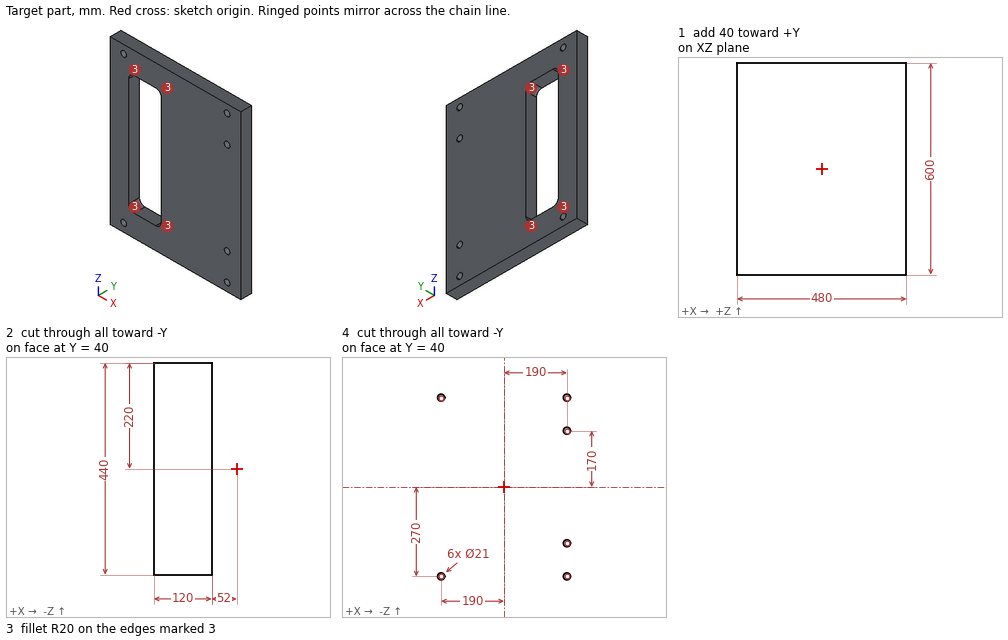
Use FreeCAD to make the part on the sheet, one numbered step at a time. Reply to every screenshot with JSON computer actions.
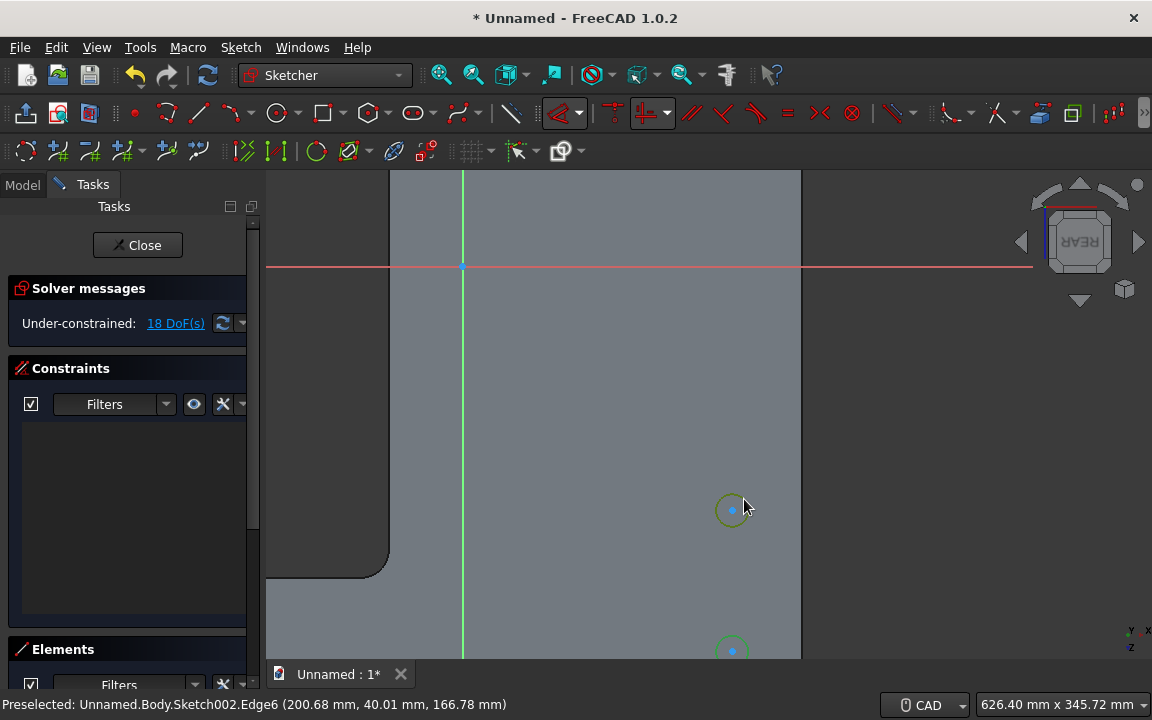
{"action": "left_click", "coordinate": [788, 114]}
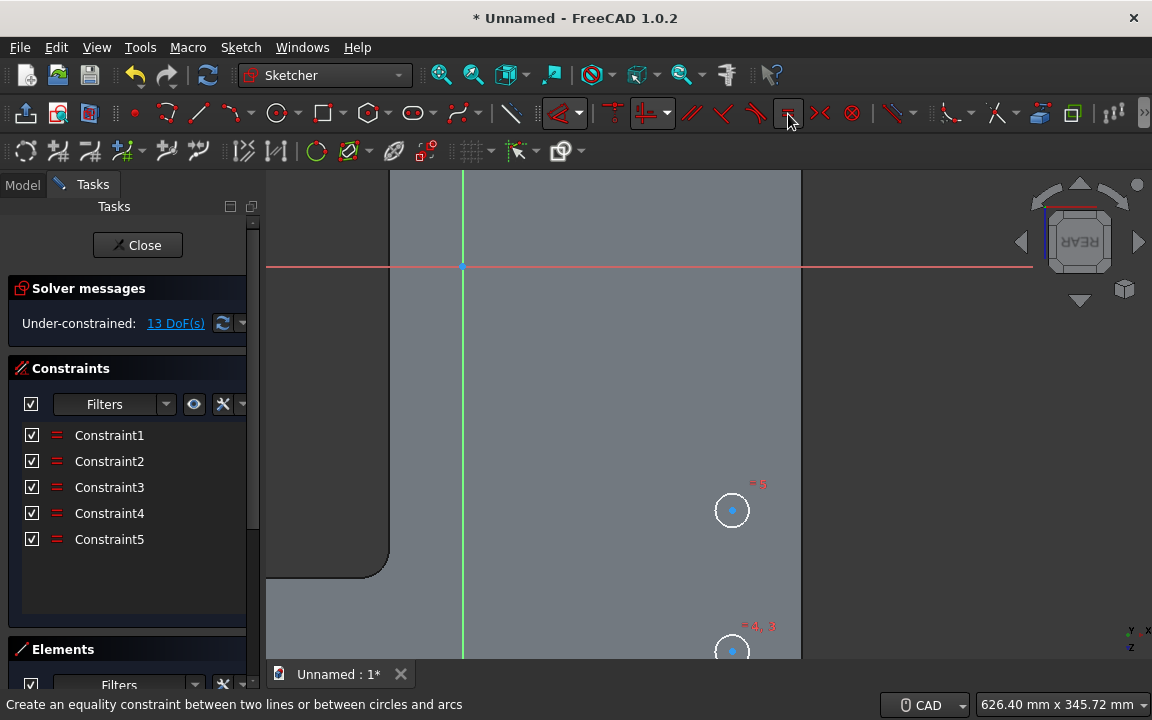
{"action": "scroll", "coordinate": [744, 500], "scroll_direction": "down", "scroll_amount": 5}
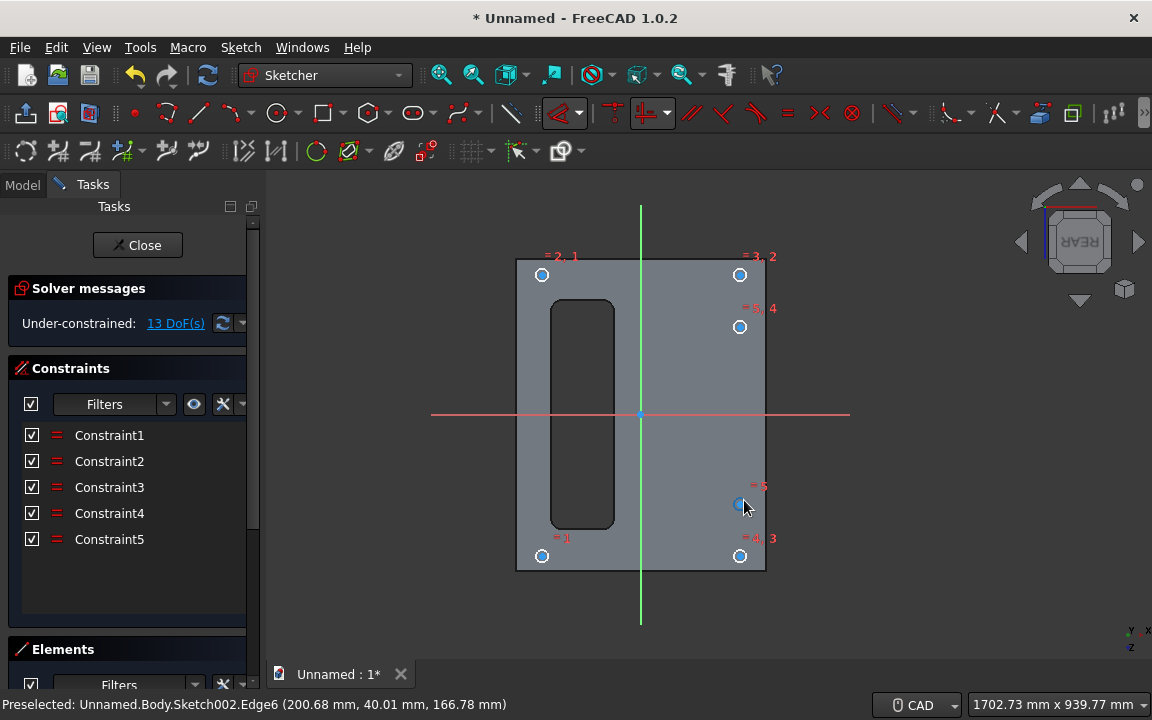
{"action": "left_click", "coordinate": [542, 556]}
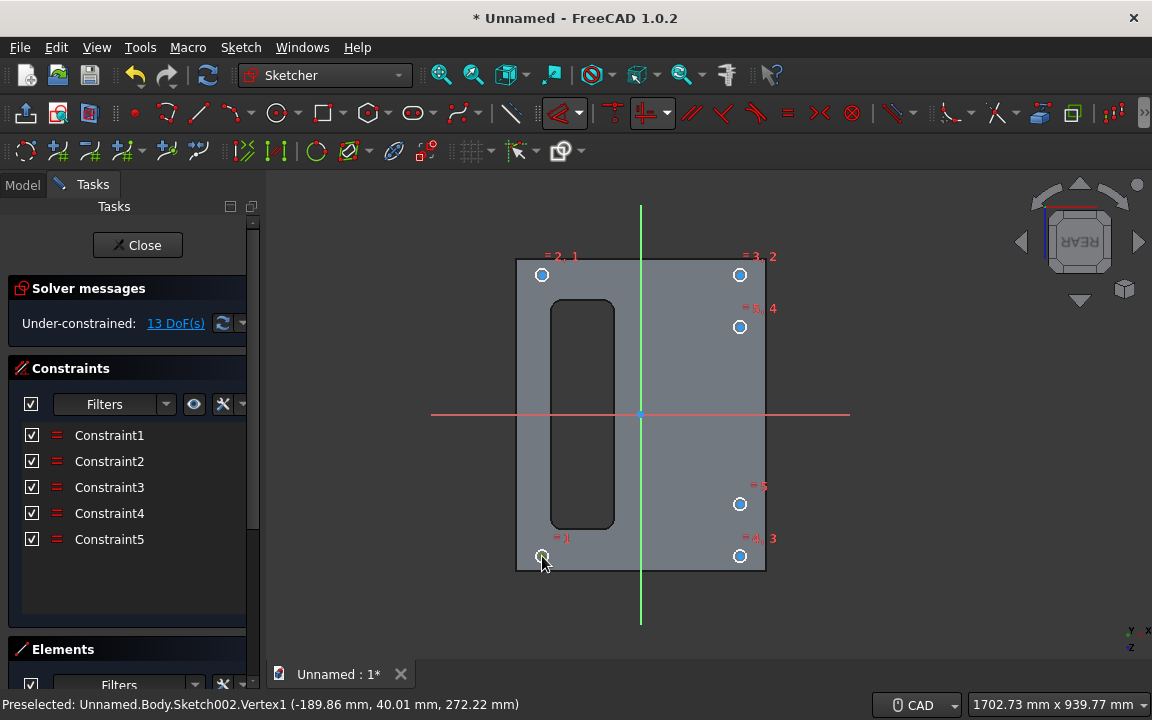
{"action": "left_click", "coordinate": [542, 275]}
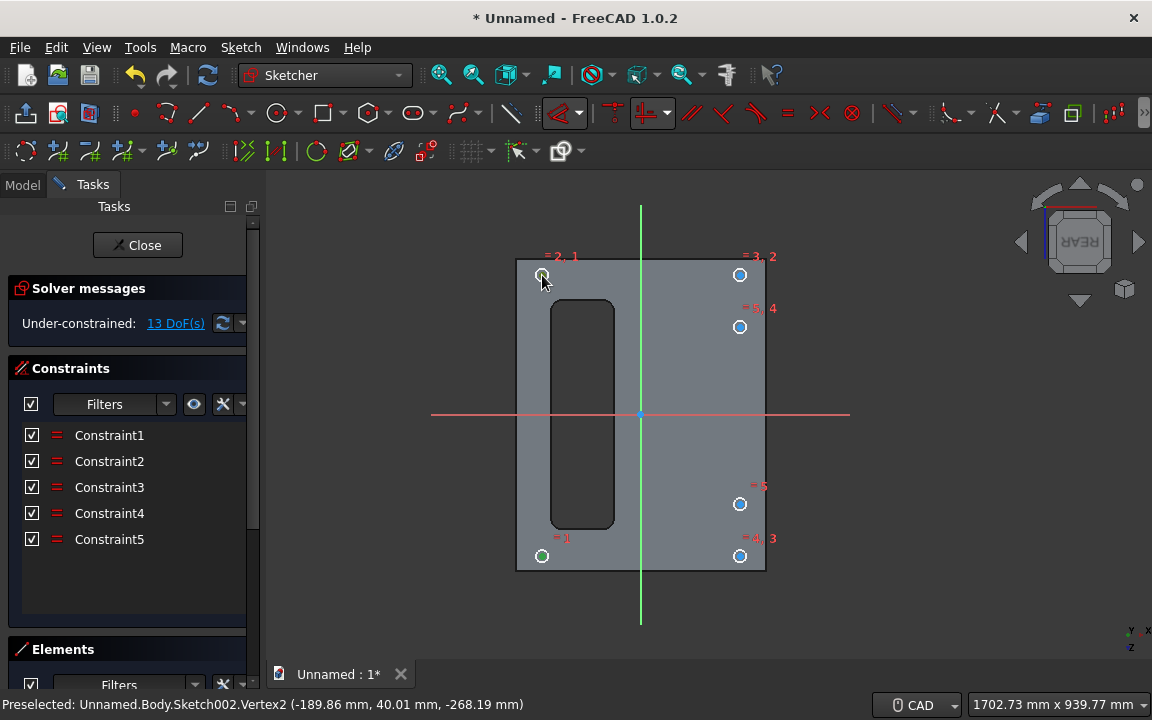
{"action": "left_click", "coordinate": [442, 415]}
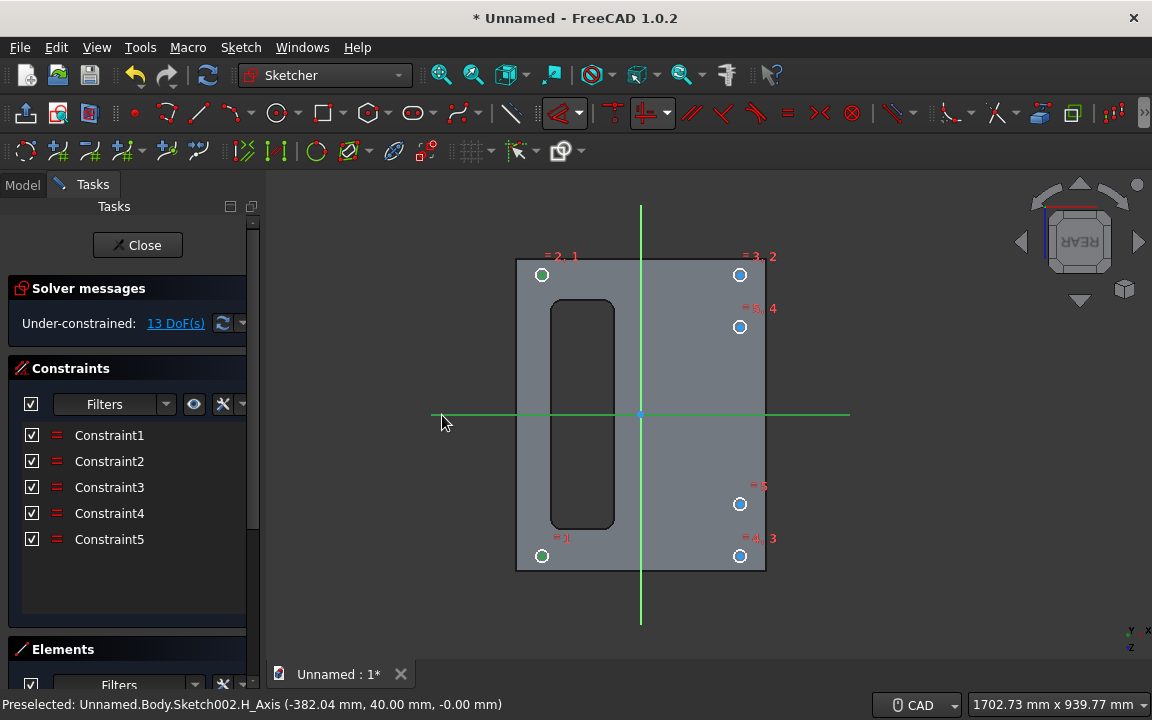
{"action": "key", "text": "s"}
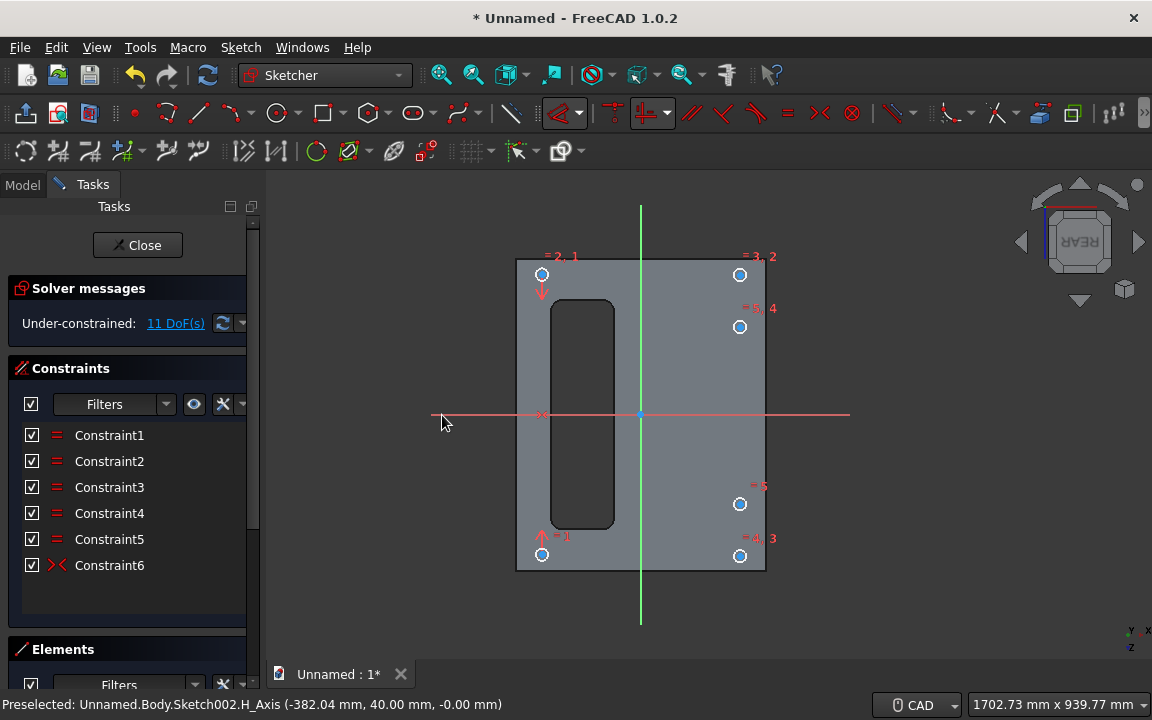
{"action": "left_click", "coordinate": [542, 275]}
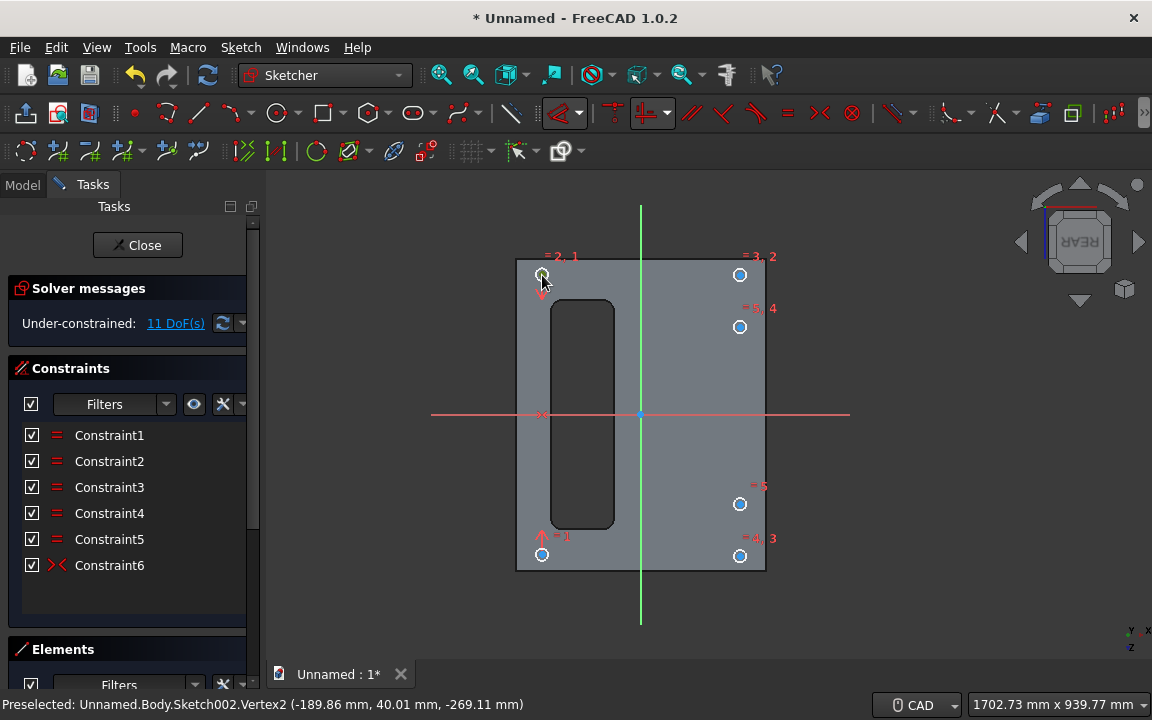
{"action": "left_click", "coordinate": [740, 275]}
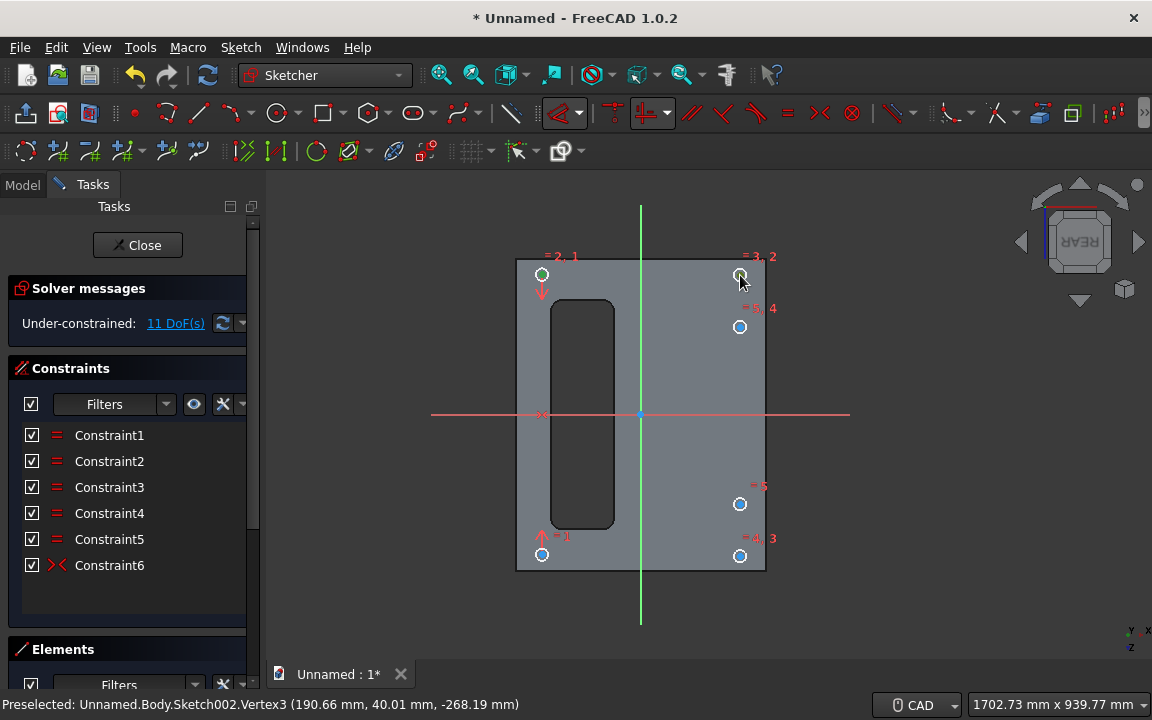
{"action": "left_click", "coordinate": [641, 600]}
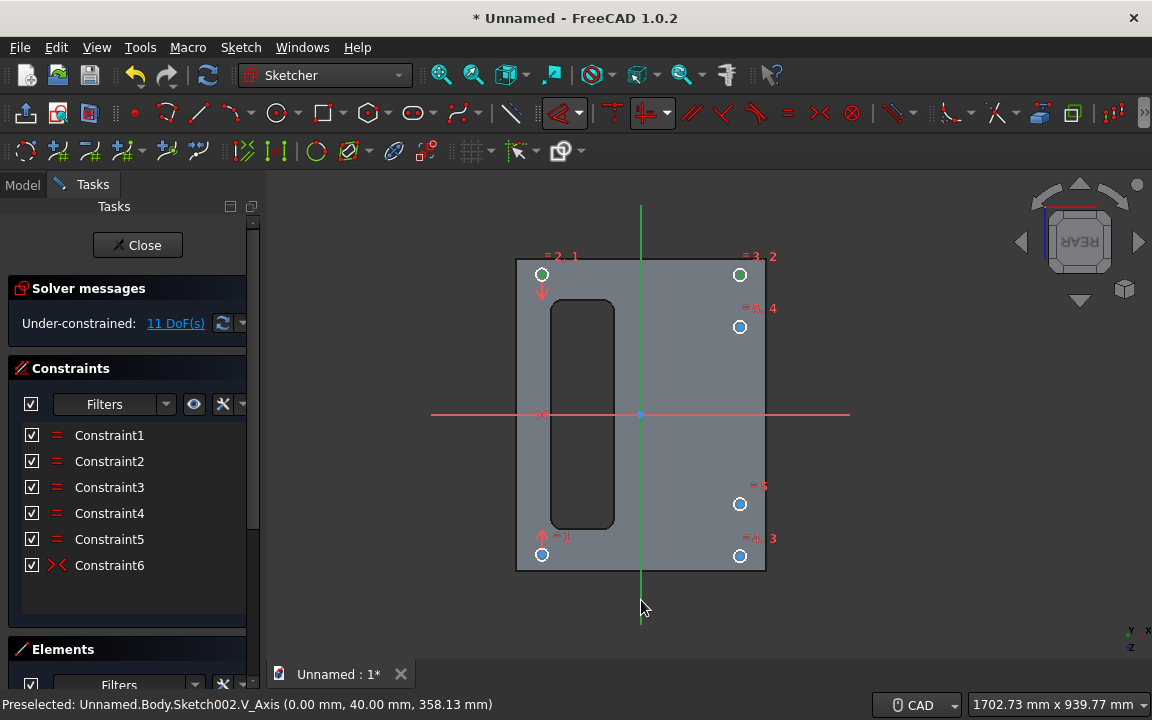
{"action": "left_click", "coordinate": [820, 114]}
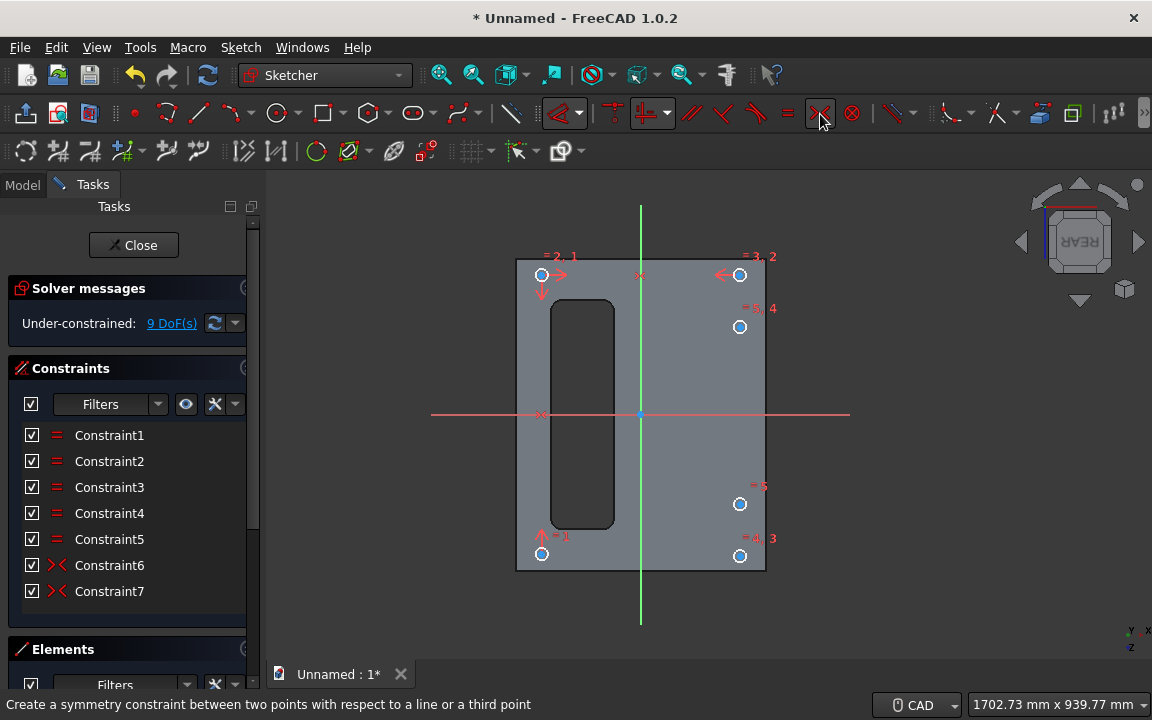
{"action": "left_click", "coordinate": [542, 554]}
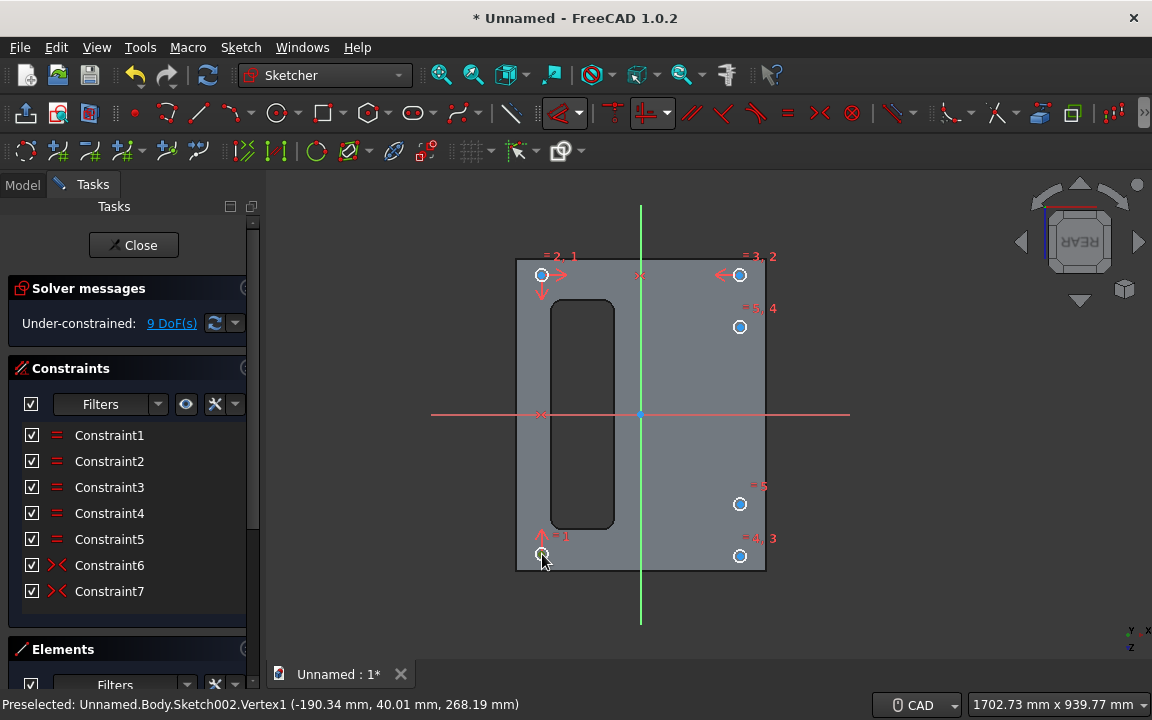
{"action": "left_click", "coordinate": [740, 556]}